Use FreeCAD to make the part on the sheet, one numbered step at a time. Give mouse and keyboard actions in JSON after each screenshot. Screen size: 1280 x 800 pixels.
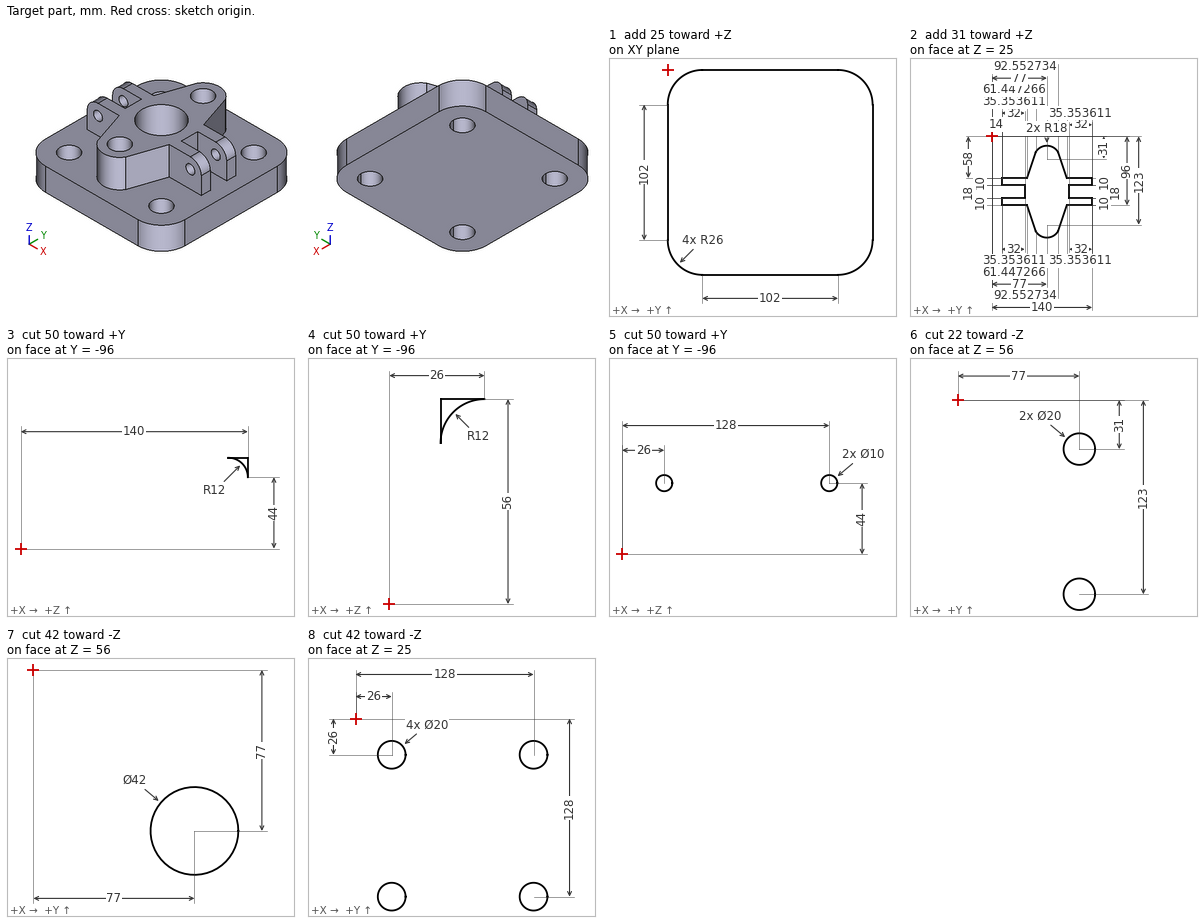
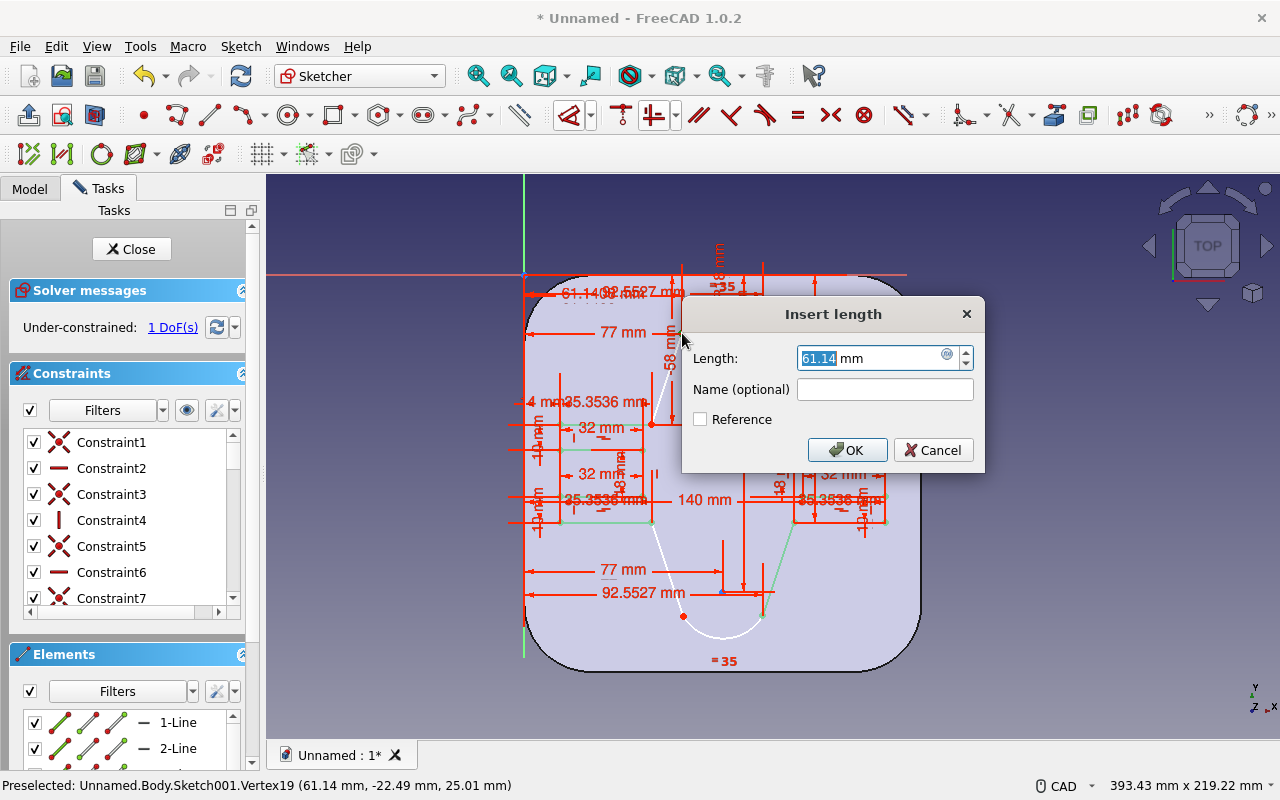
{"action": "type", "text": "61.447266"}
{"action": "key", "text": "Return"}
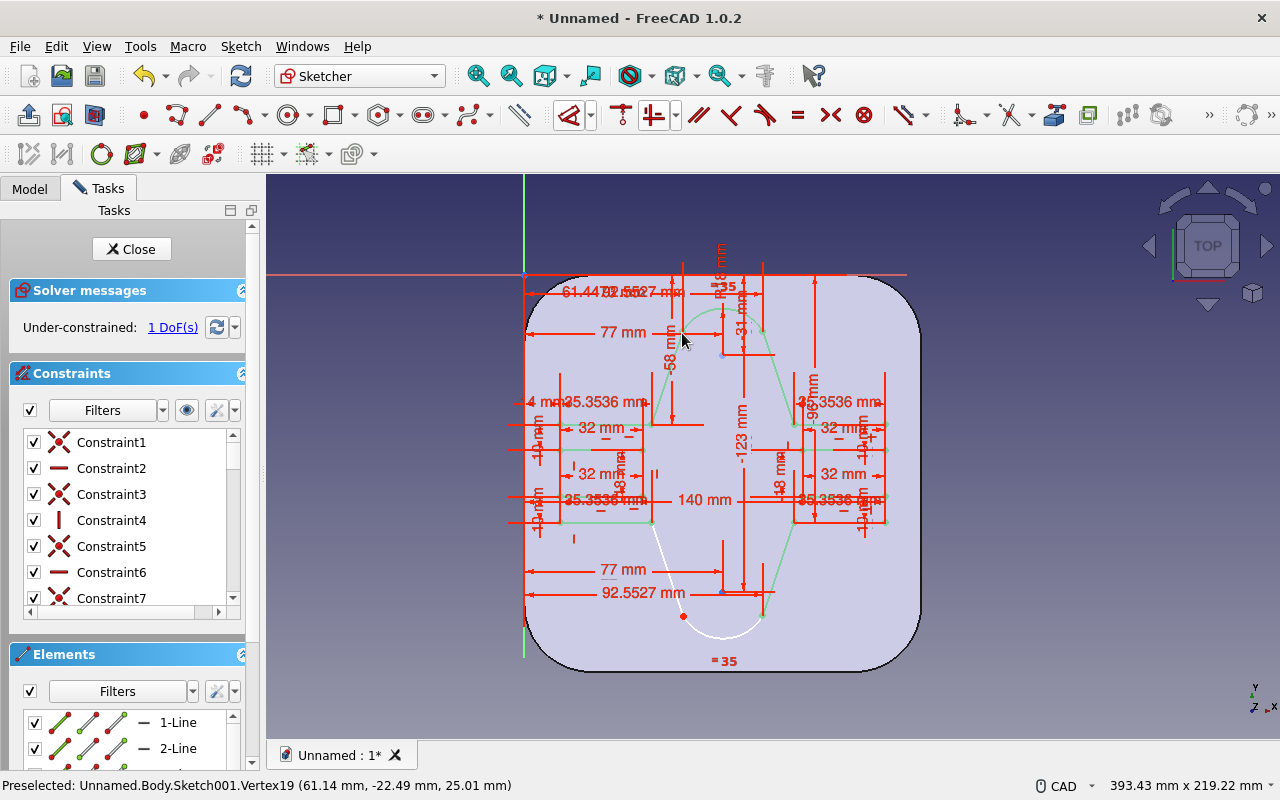
{"action": "left_click", "coordinate": [683, 616]}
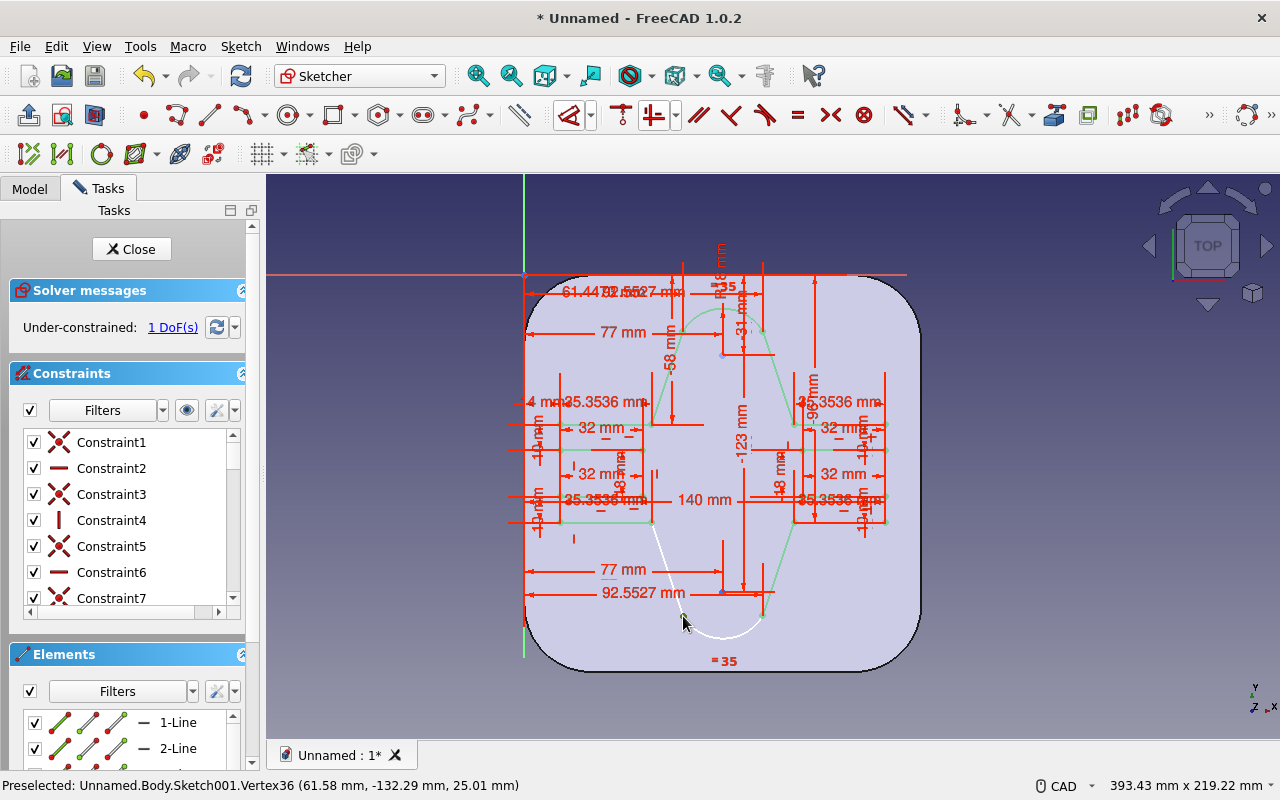
{"action": "left_click", "coordinate": [590, 116]}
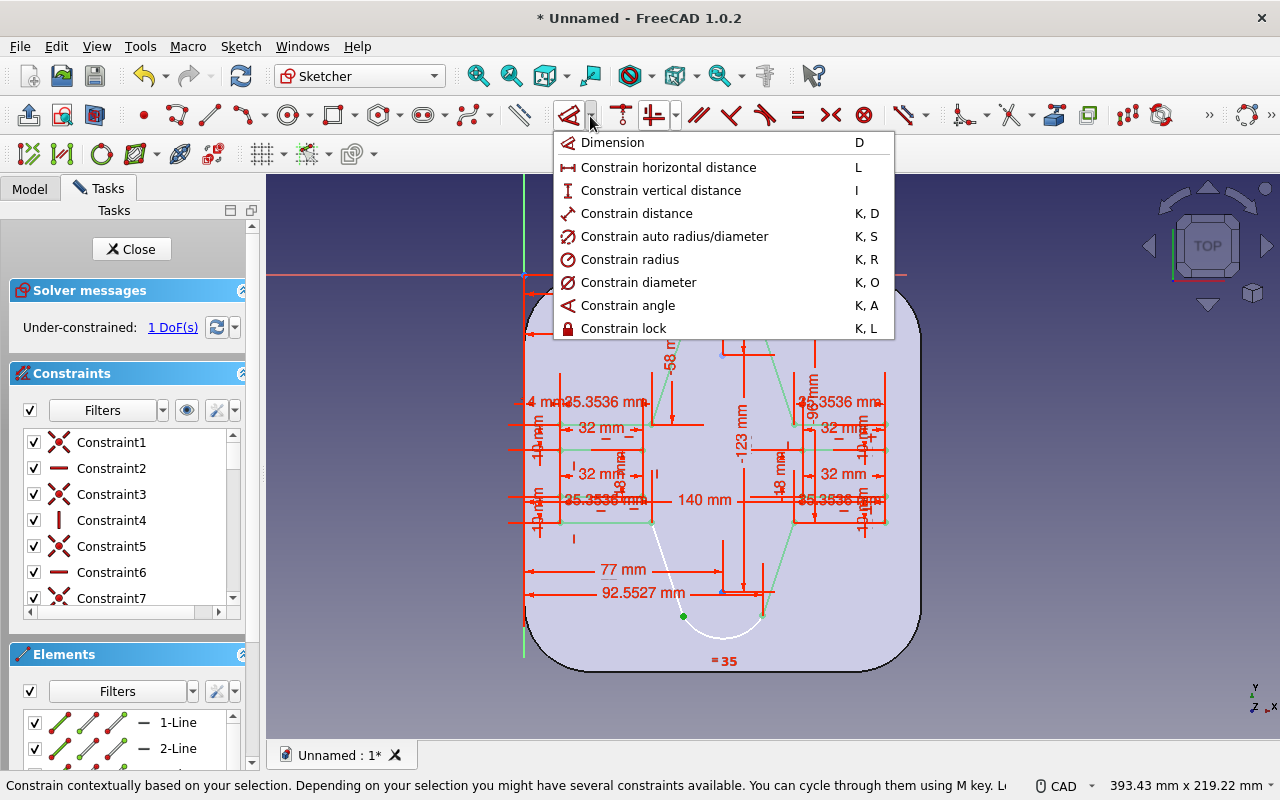
{"action": "left_click", "coordinate": [724, 168]}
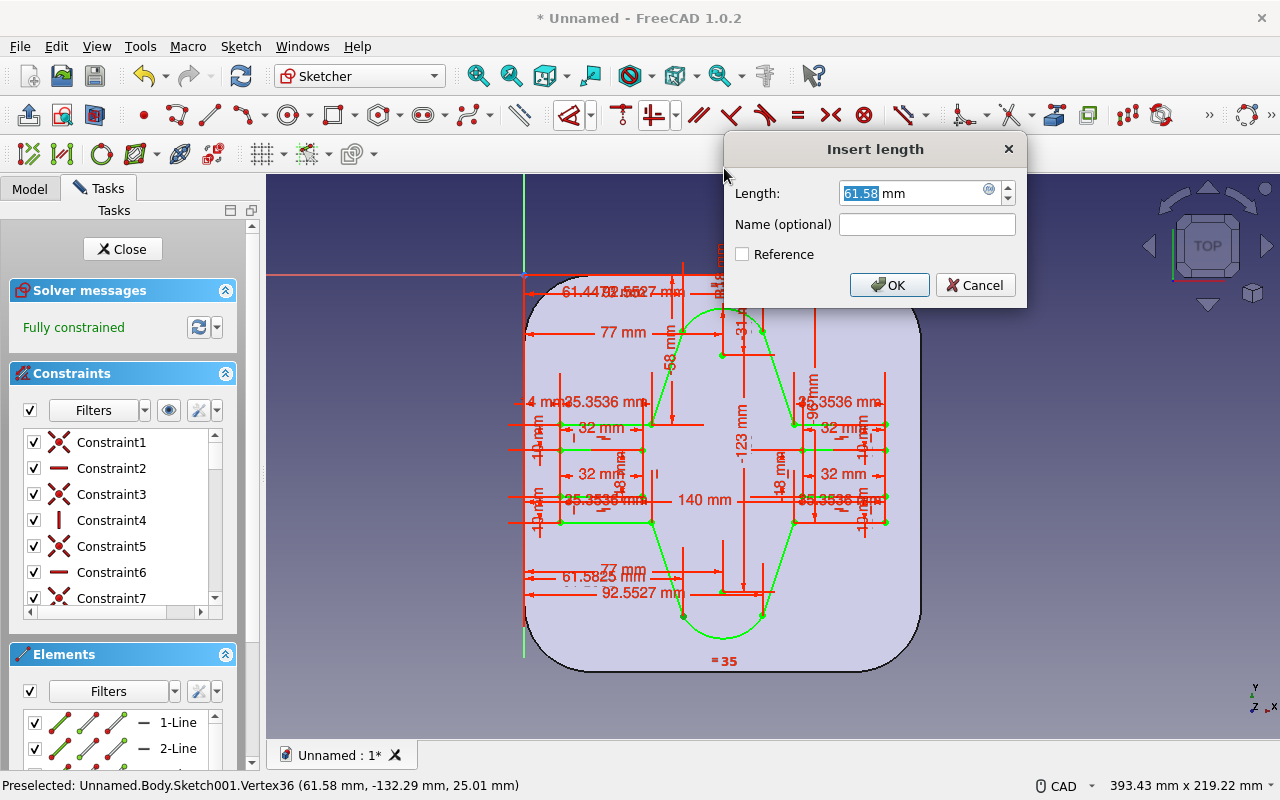
{"action": "type", "text": "61.447266"}
{"action": "key", "text": "Return"}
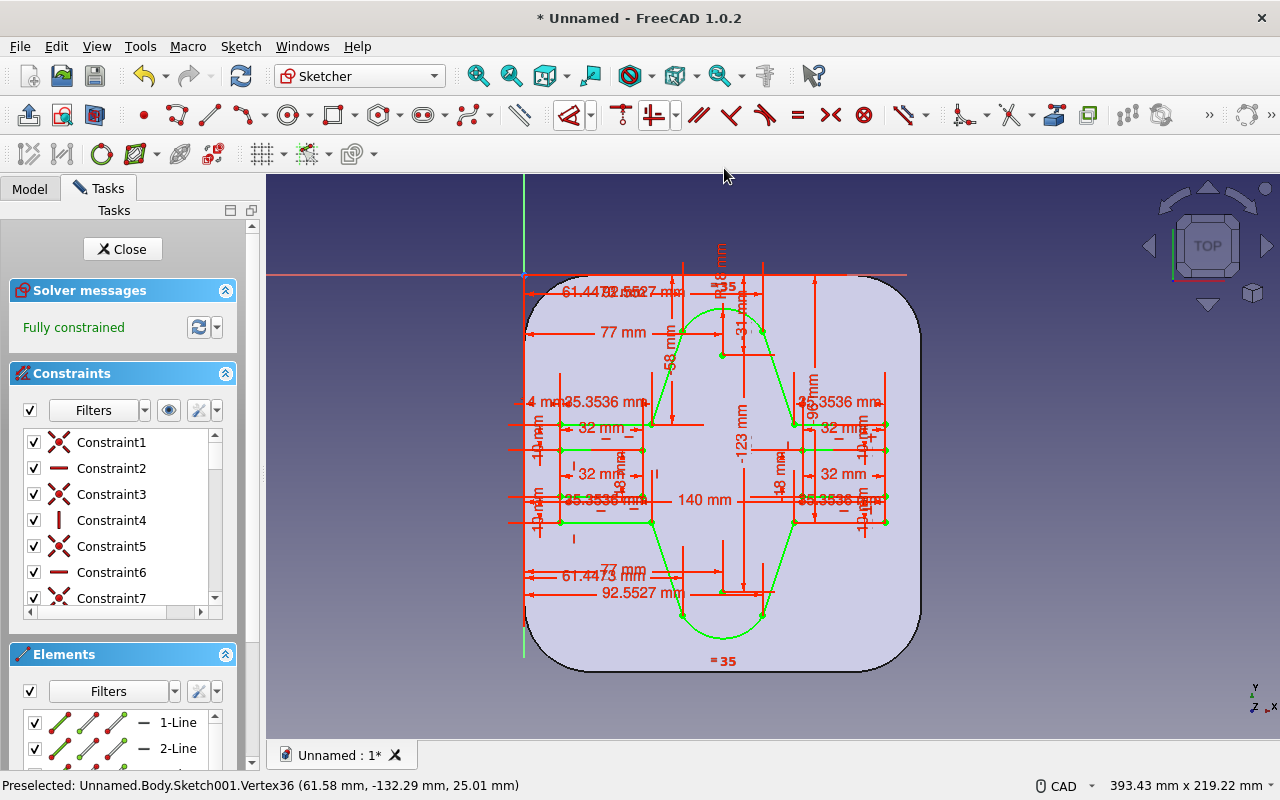
{"action": "left_click", "coordinate": [123, 249]}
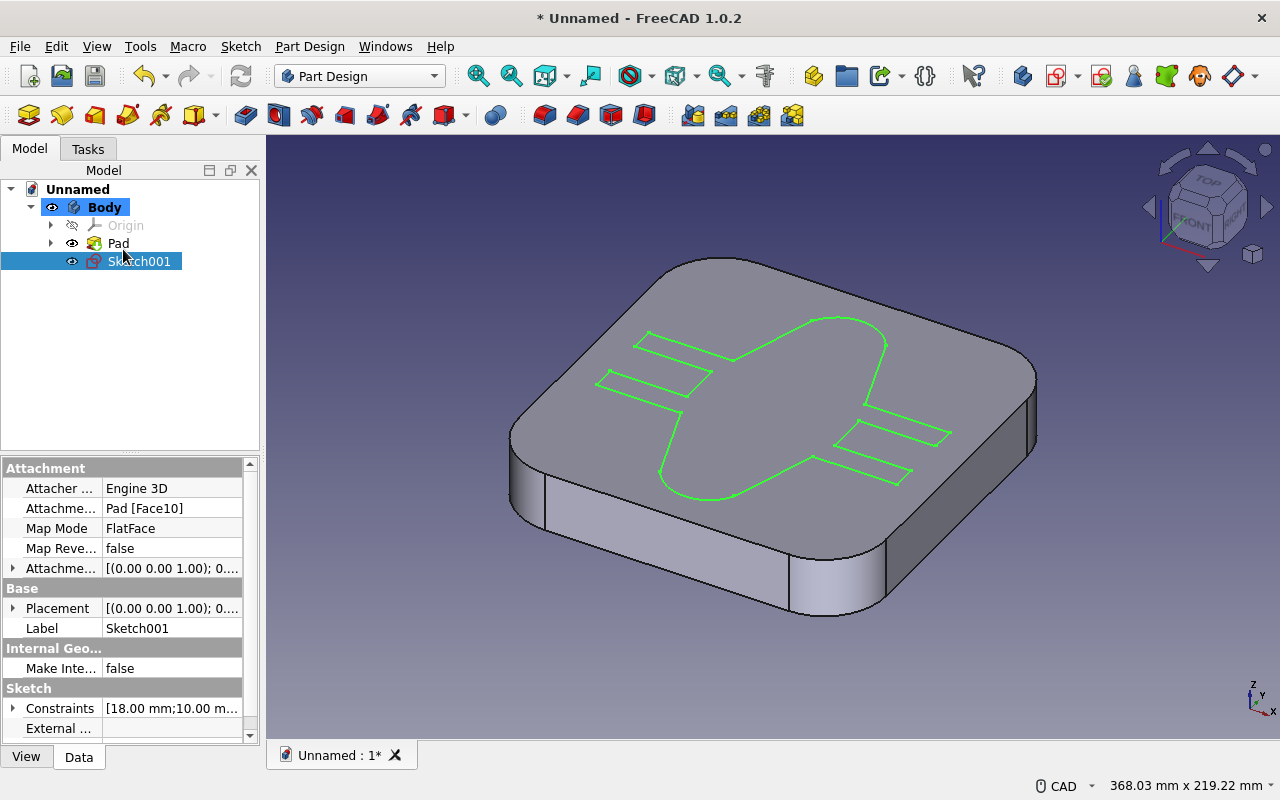
{"action": "left_click", "coordinate": [29, 116]}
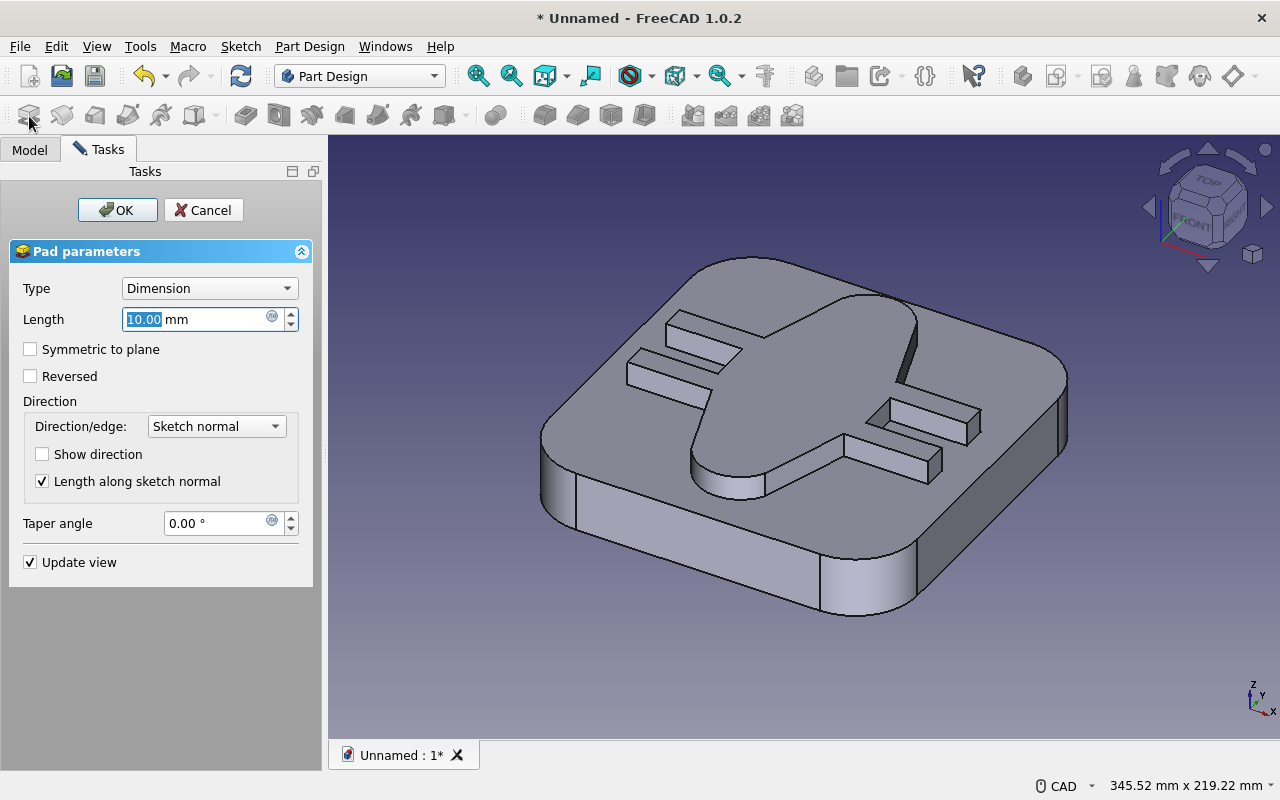
{"action": "type", "text": "31"}
{"action": "key", "text": "Tab"}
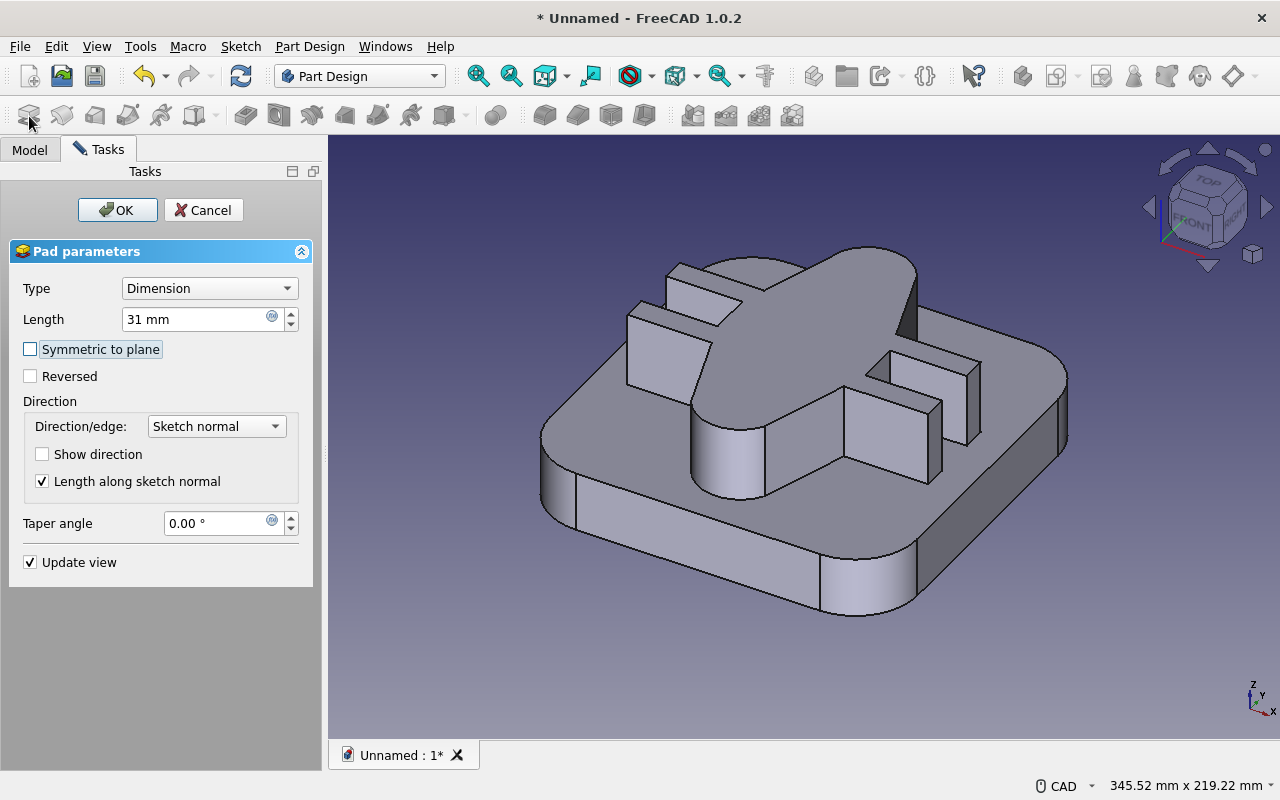
{"action": "left_click", "coordinate": [118, 210]}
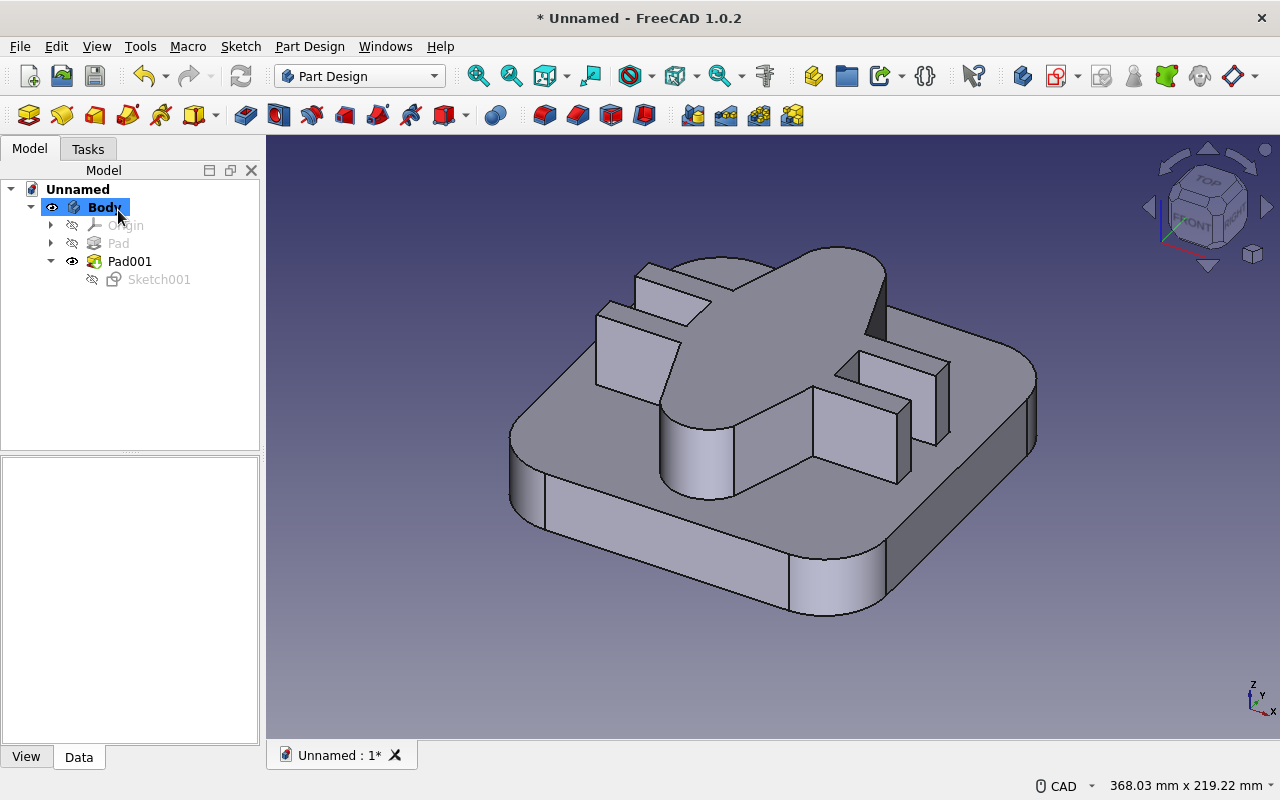
{"action": "left_click", "coordinate": [639, 363]}